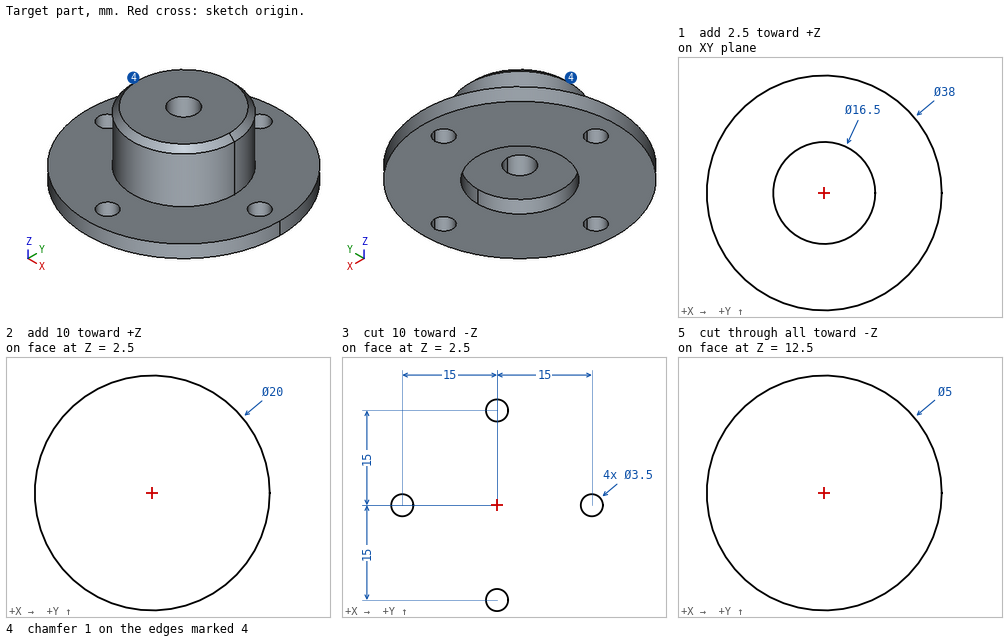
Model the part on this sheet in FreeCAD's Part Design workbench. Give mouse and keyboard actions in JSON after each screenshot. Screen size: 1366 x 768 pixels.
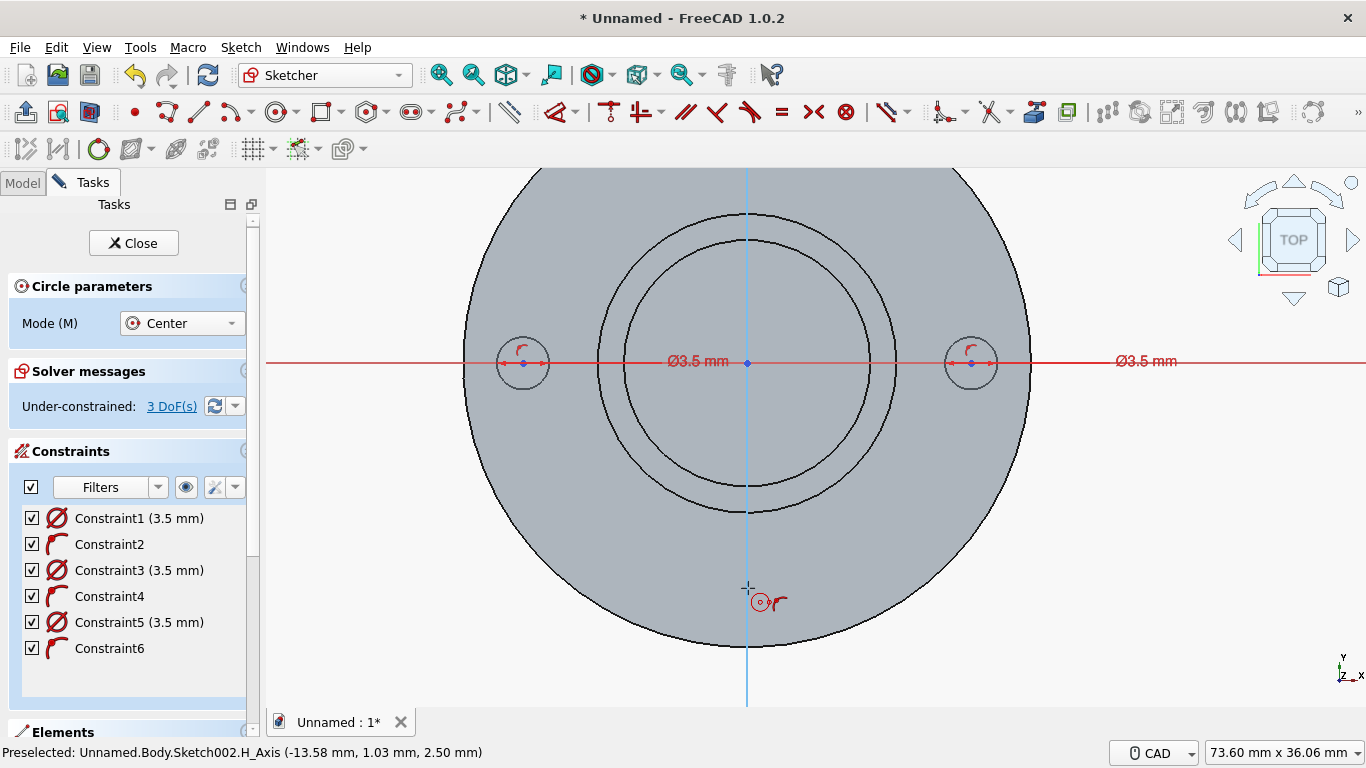
{"action": "left_click", "coordinate": [747, 588]}
{"action": "mouse_move", "coordinate": [766, 569]}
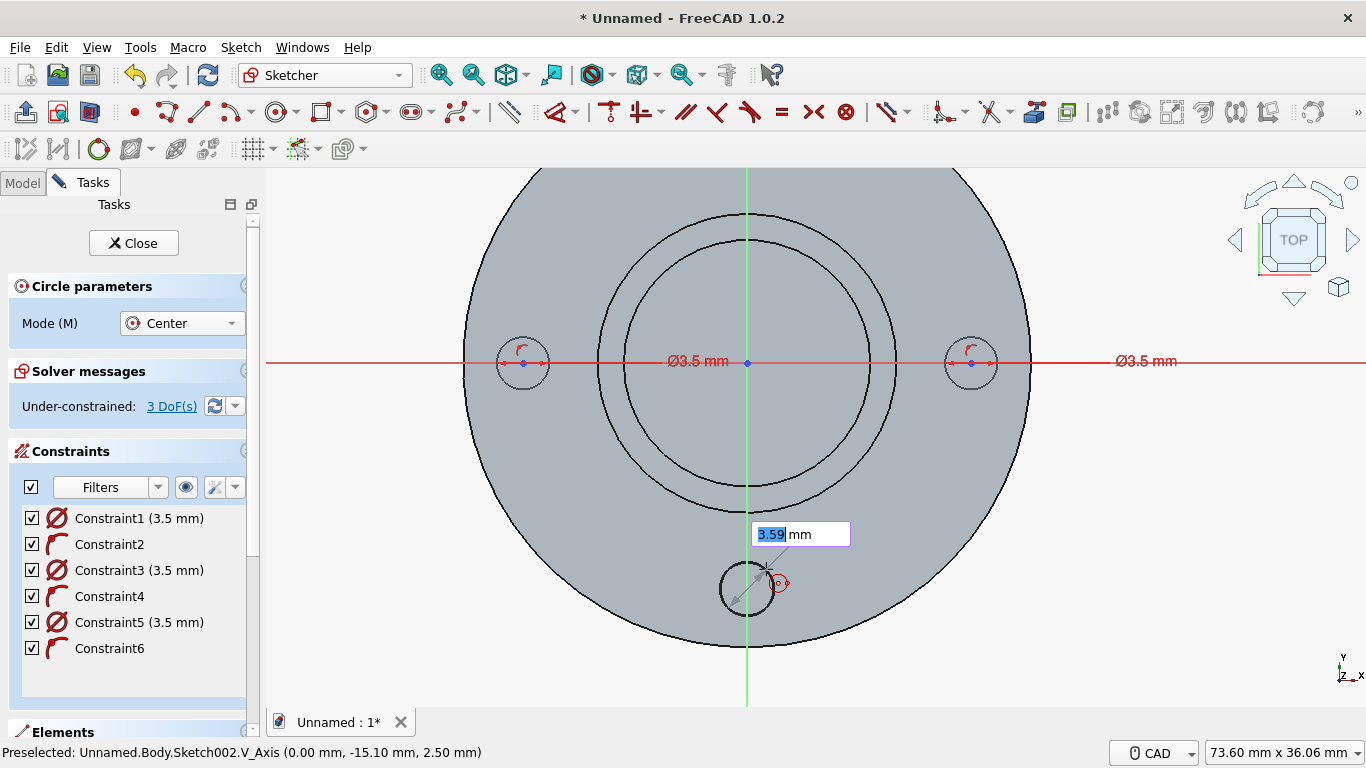
{"action": "type", "text": "3.5"}
{"action": "key", "text": "Return"}
{"action": "key", "text": "Escape"}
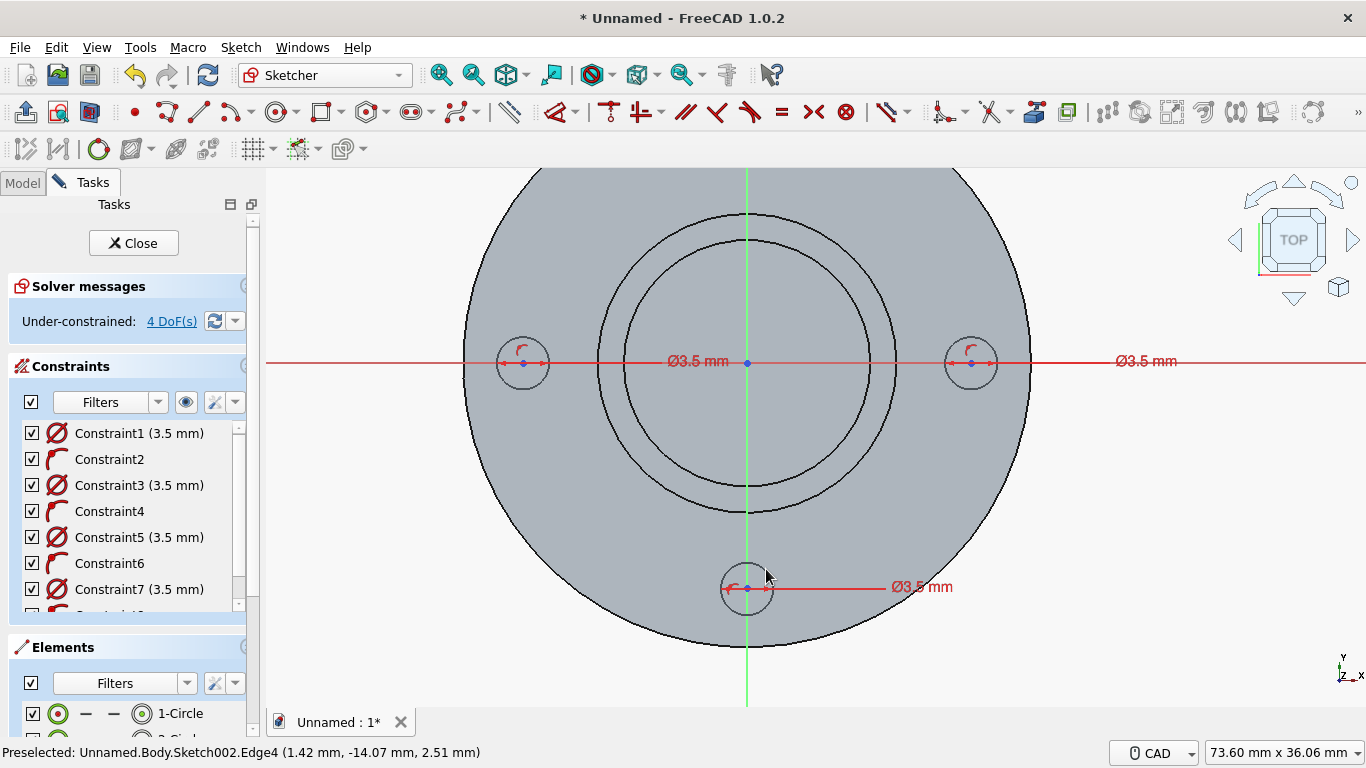
{"action": "left_click", "coordinate": [556, 112]}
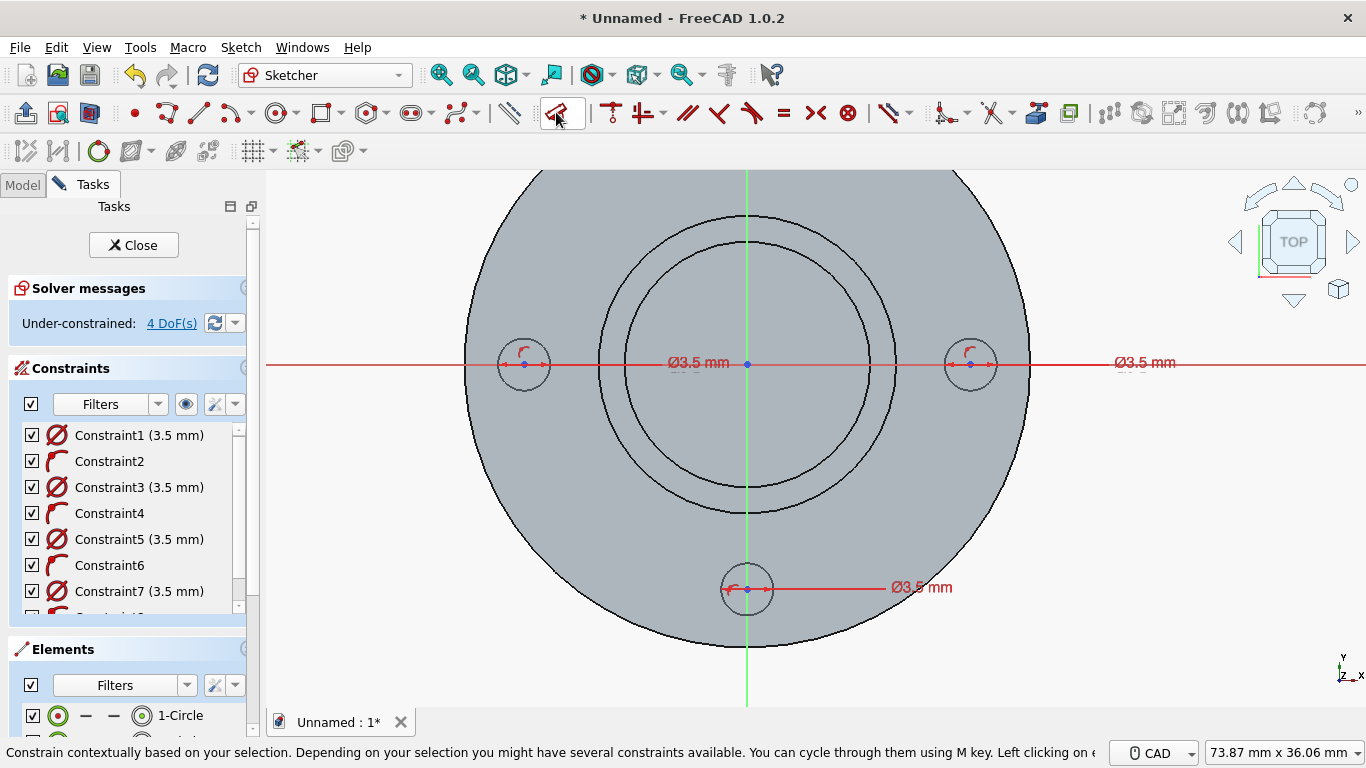
{"action": "left_click", "coordinate": [971, 365]}
{"action": "left_click", "coordinate": [859, 399]}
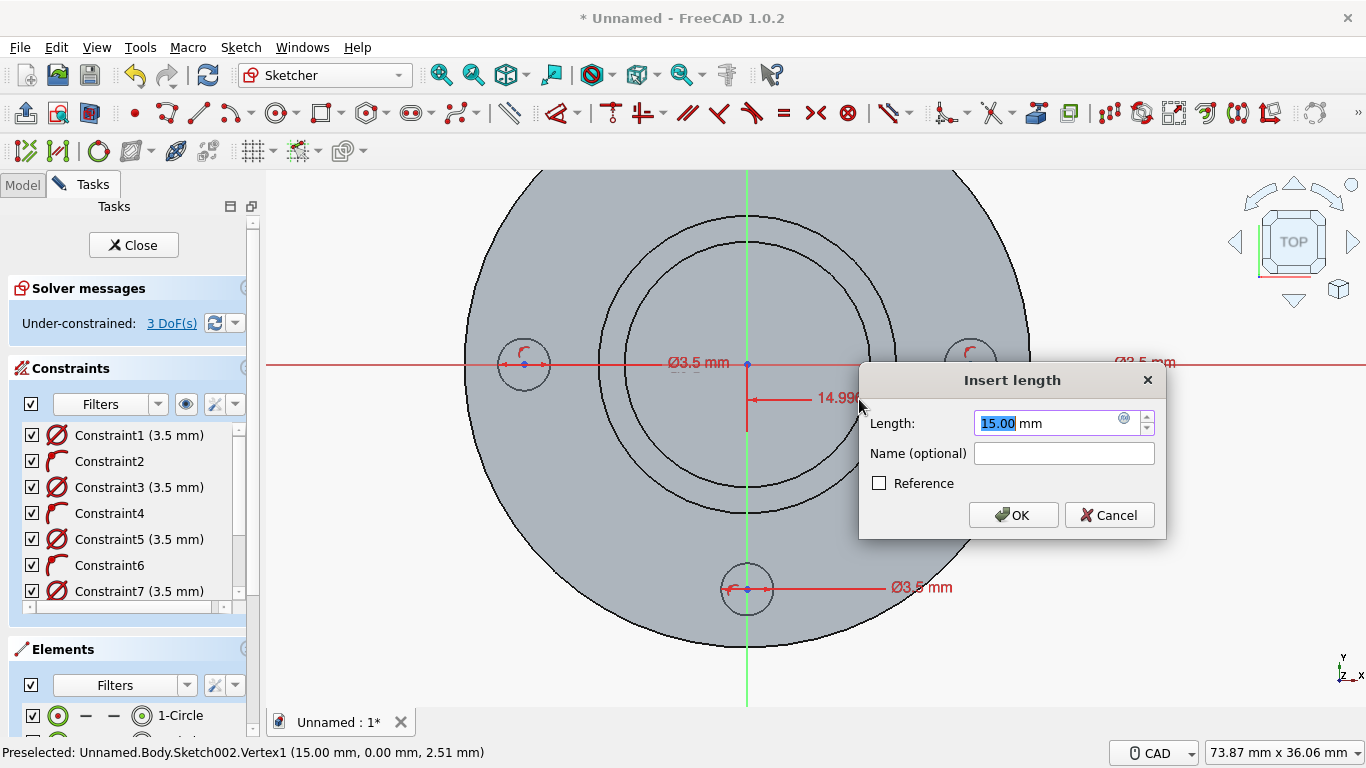
{"action": "type", "text": "15"}
{"action": "key", "text": "Return"}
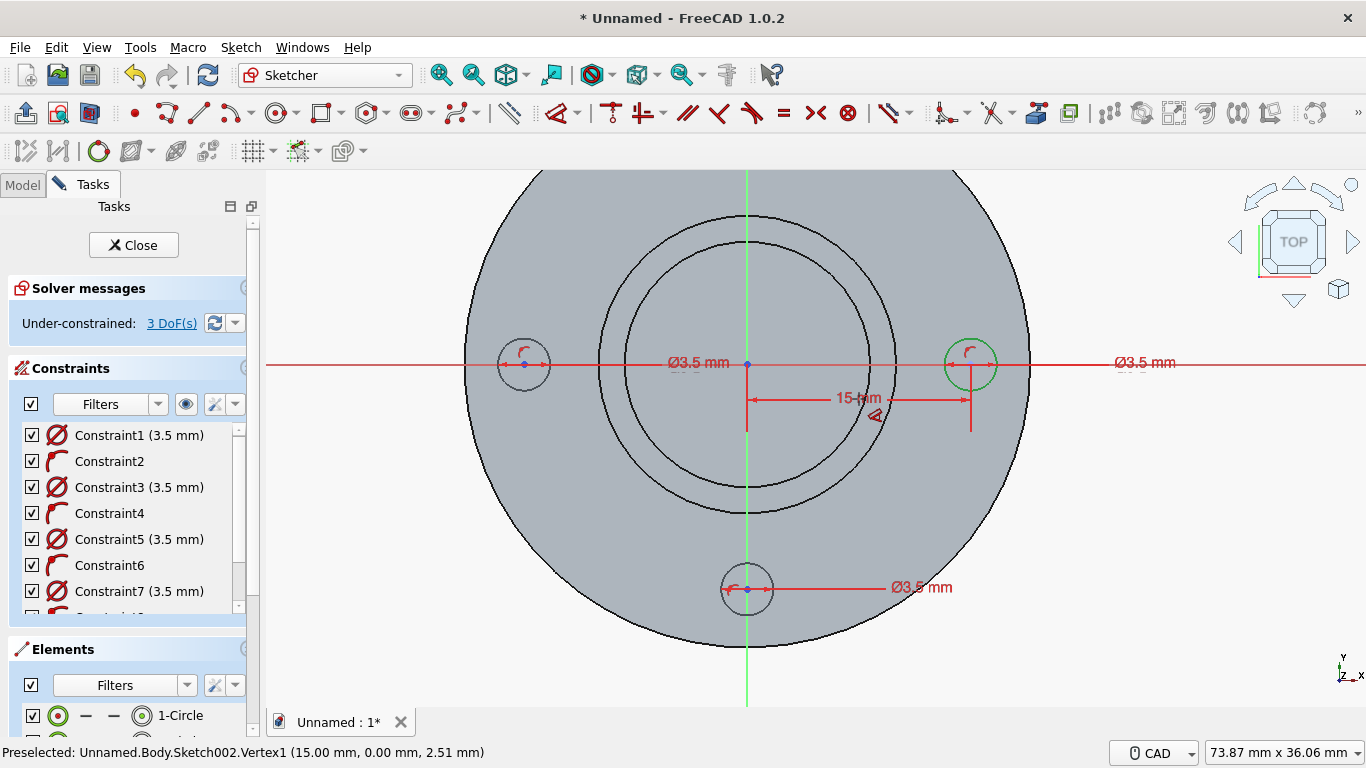
{"action": "scroll", "coordinate": [748, 589], "scroll_direction": "down", "scroll_amount": 2}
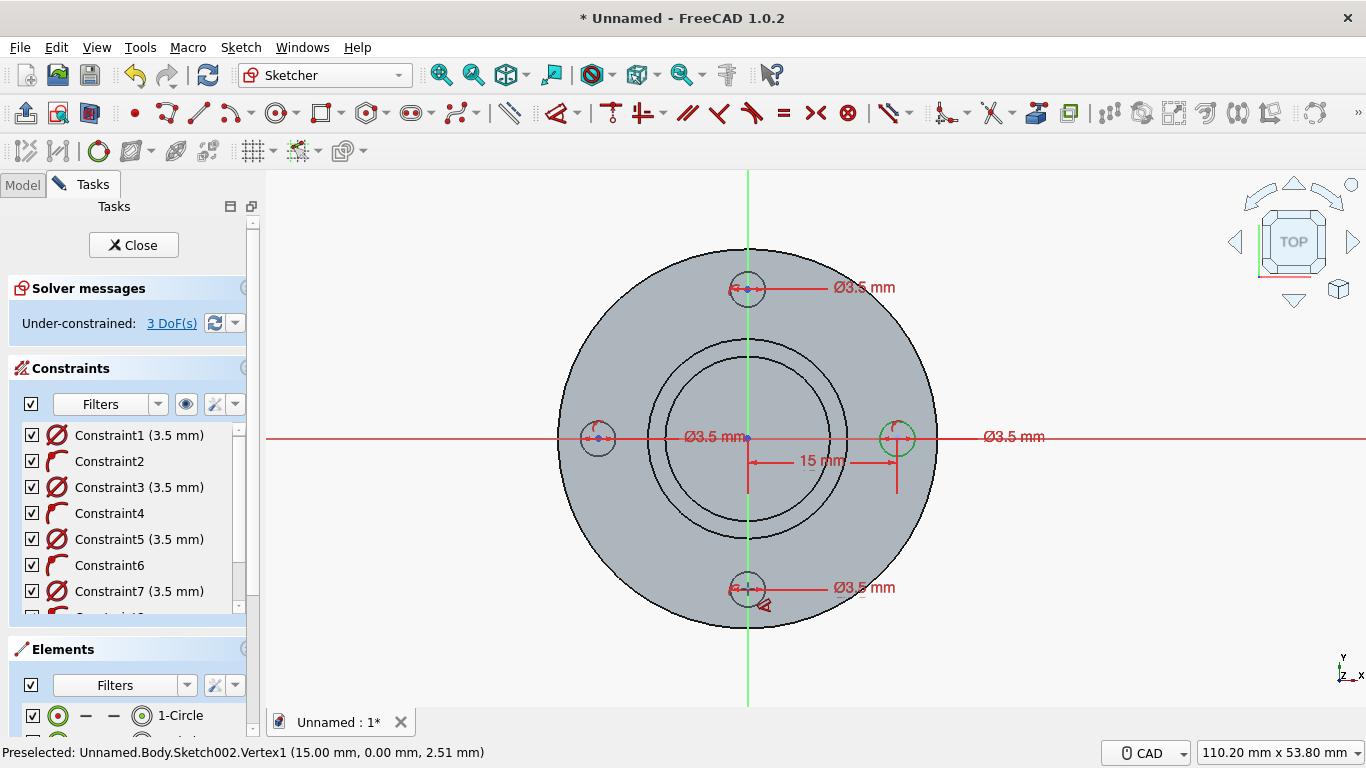
{"action": "left_click", "coordinate": [748, 289]}
{"action": "left_click", "coordinate": [782, 364]}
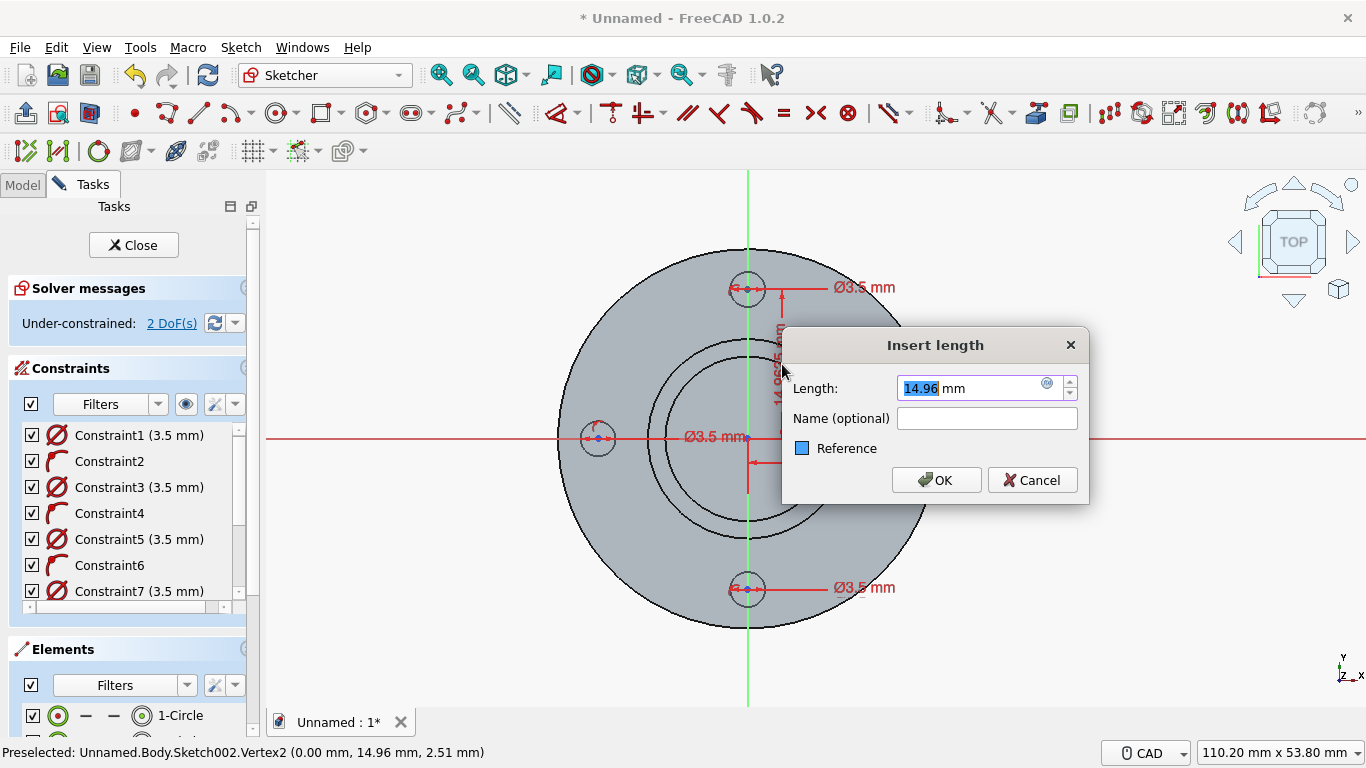
{"action": "type", "text": "15"}
{"action": "key", "text": "Return"}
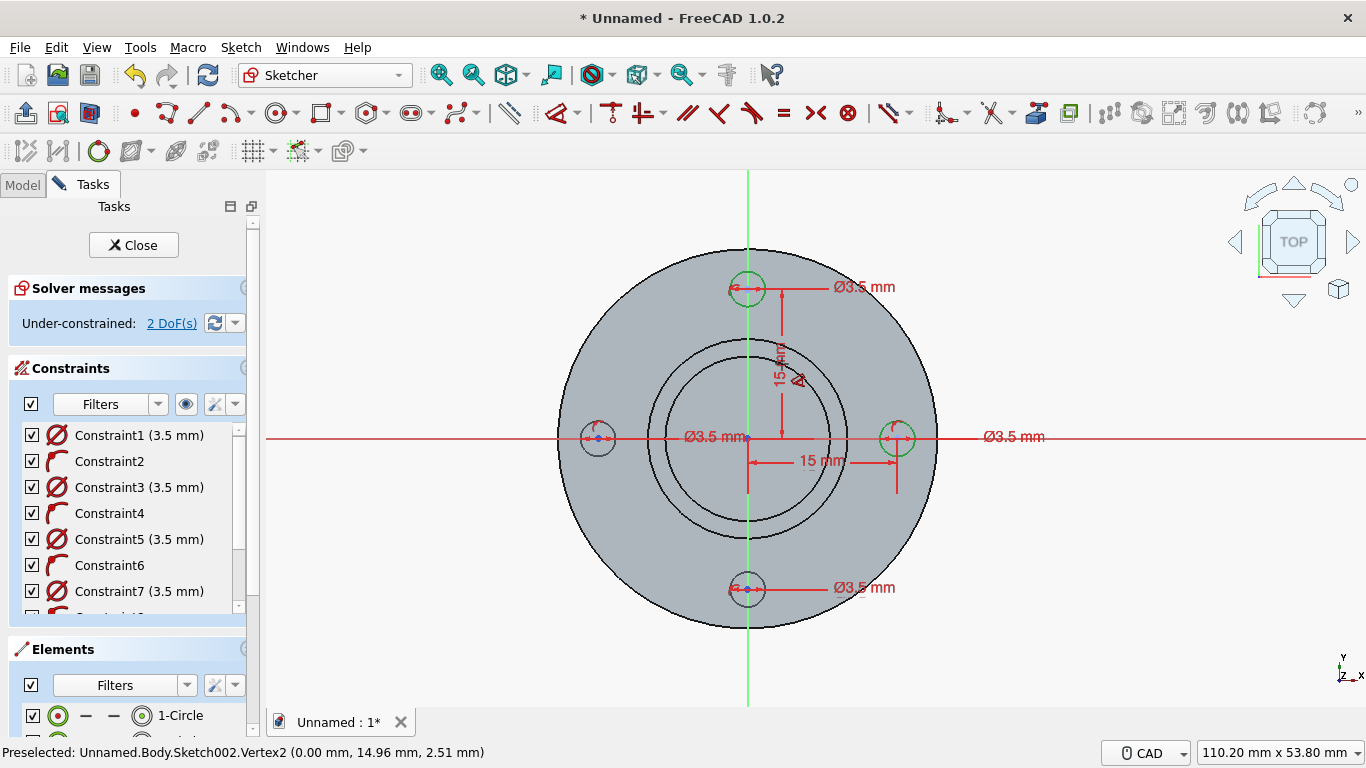
{"action": "left_click", "coordinate": [598, 439]}
{"action": "left_click", "coordinate": [673, 473]}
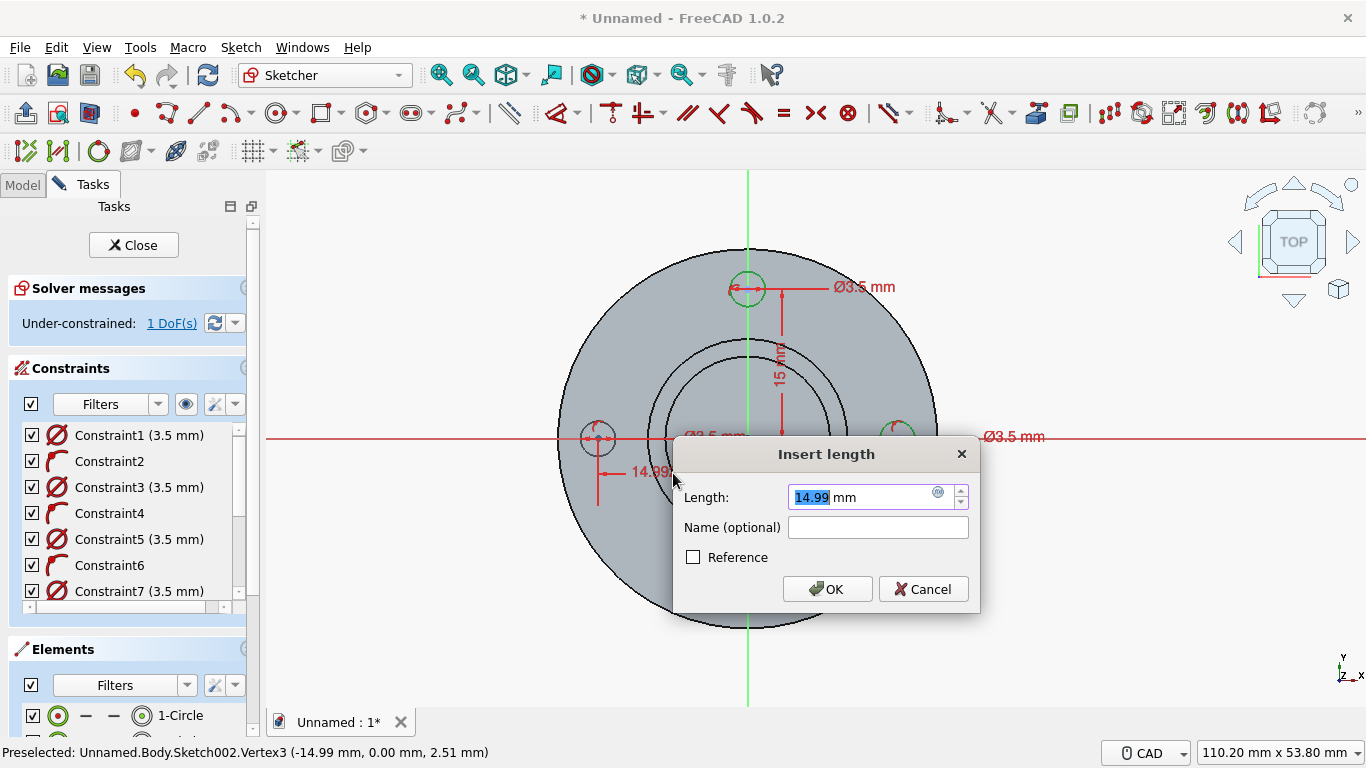
{"action": "type", "text": "15"}
{"action": "key", "text": "Return"}